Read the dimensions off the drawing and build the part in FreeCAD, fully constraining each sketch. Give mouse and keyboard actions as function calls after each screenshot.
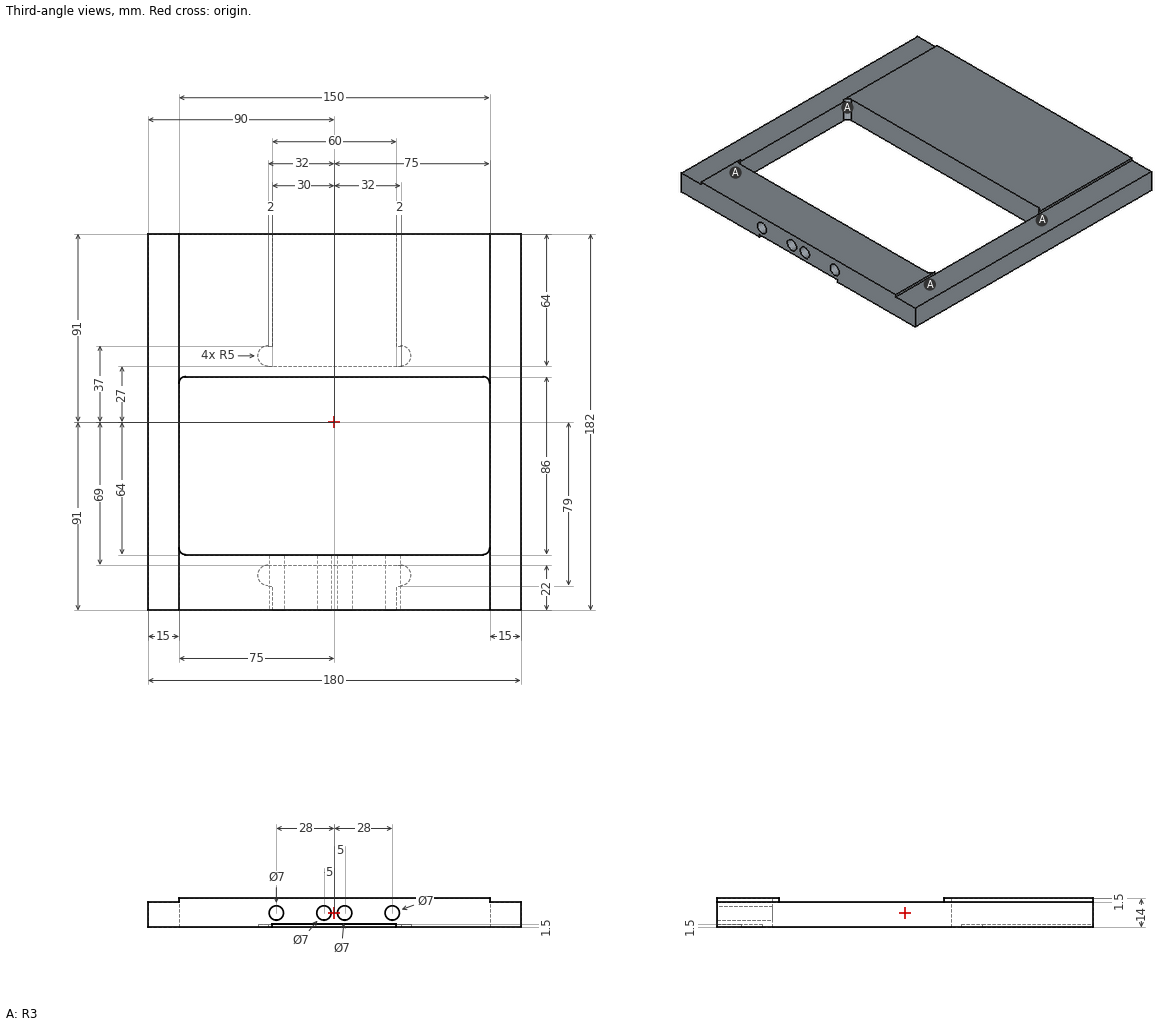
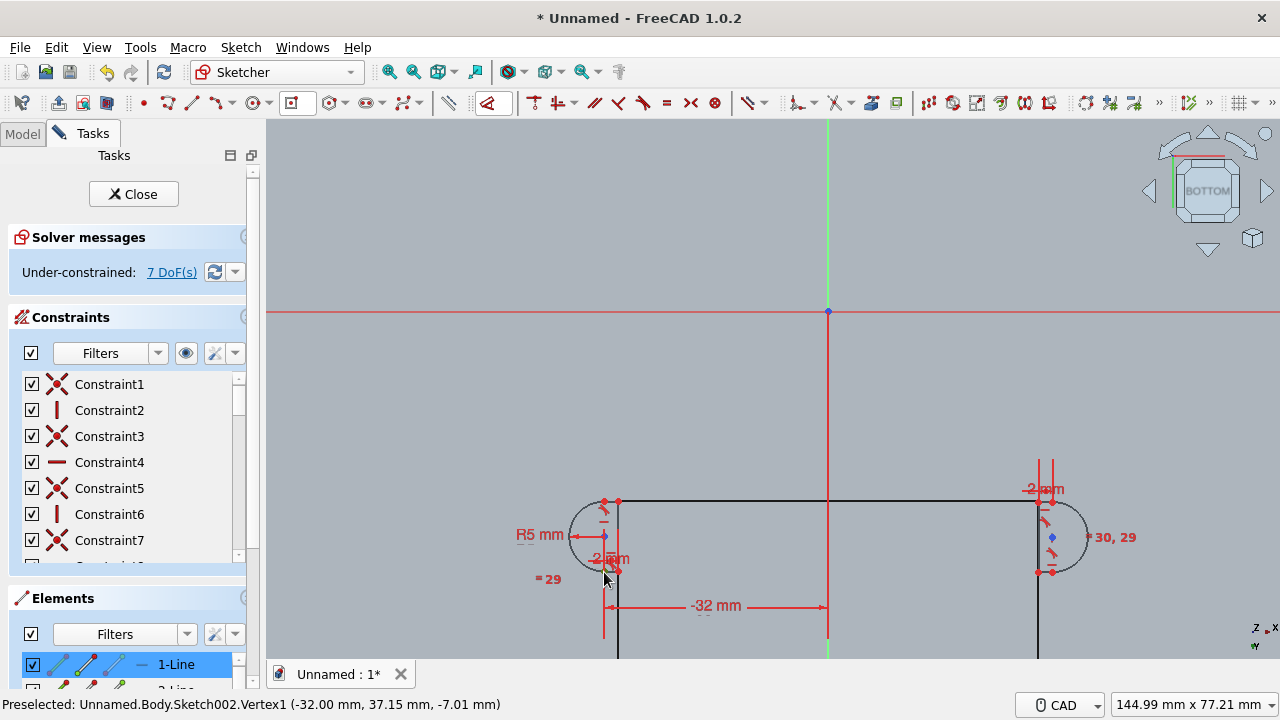
key(i)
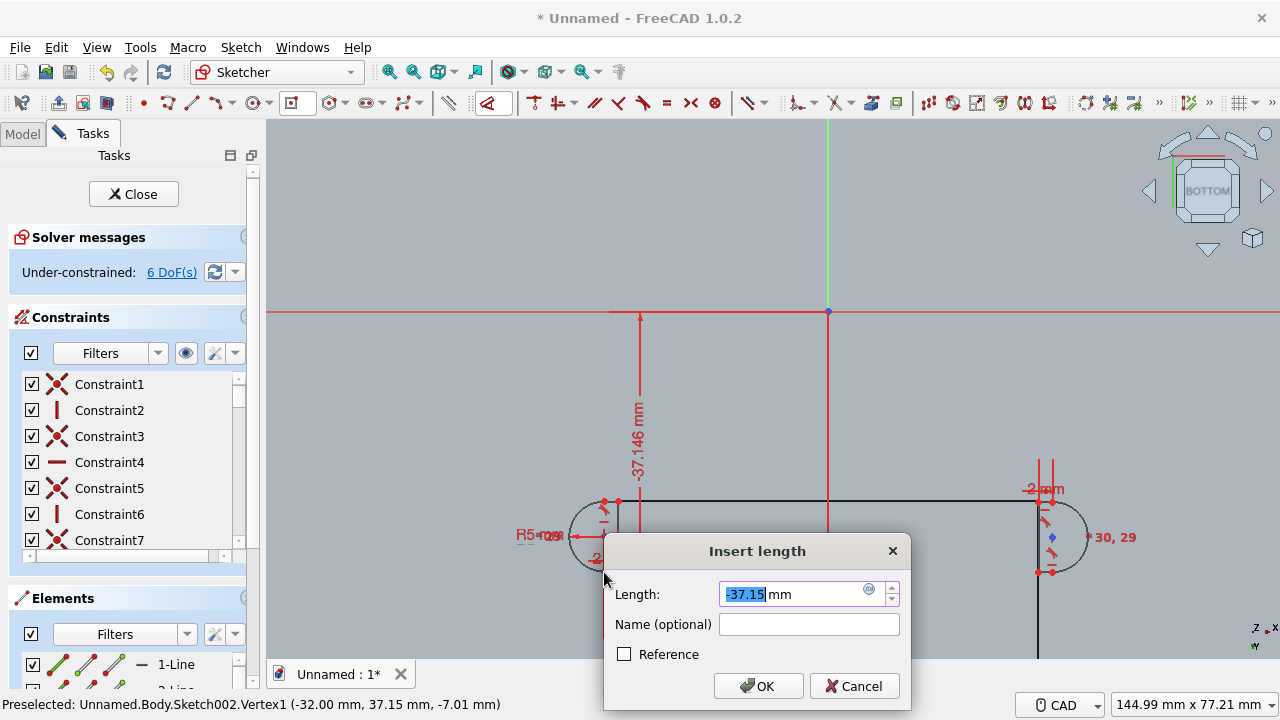
text(-37)
key(Return)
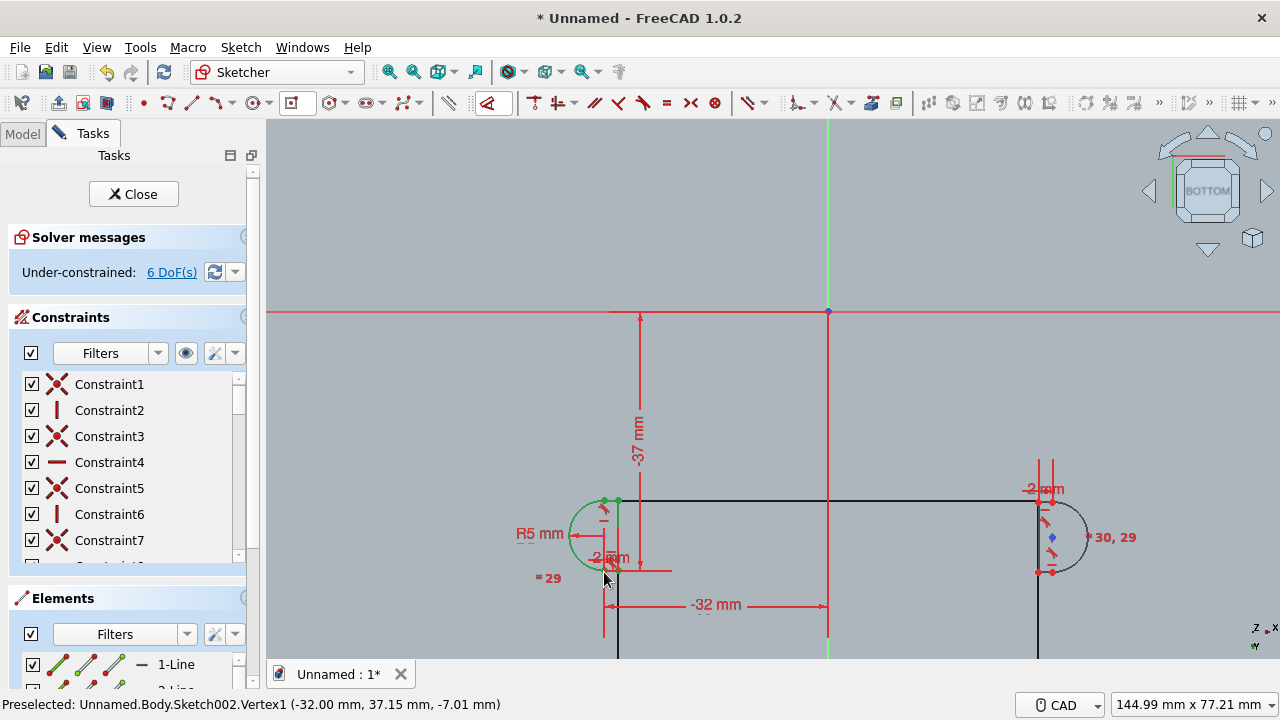
click(1053, 502)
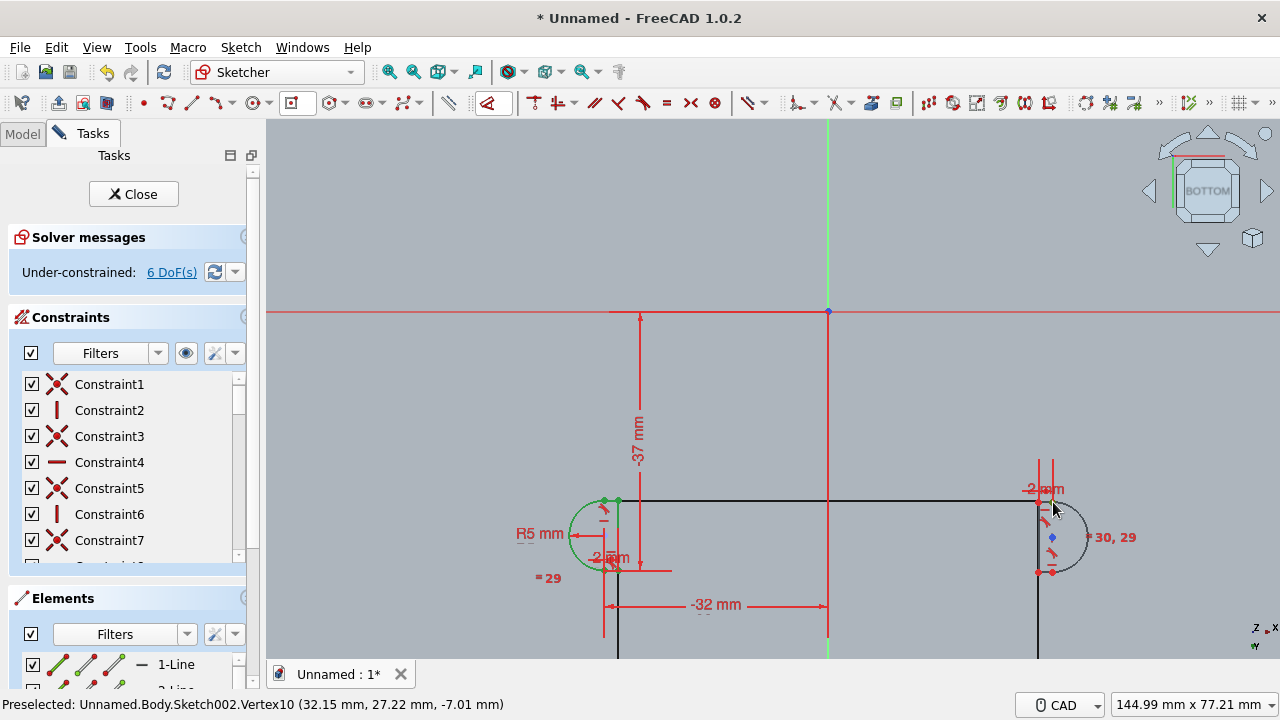
key(l)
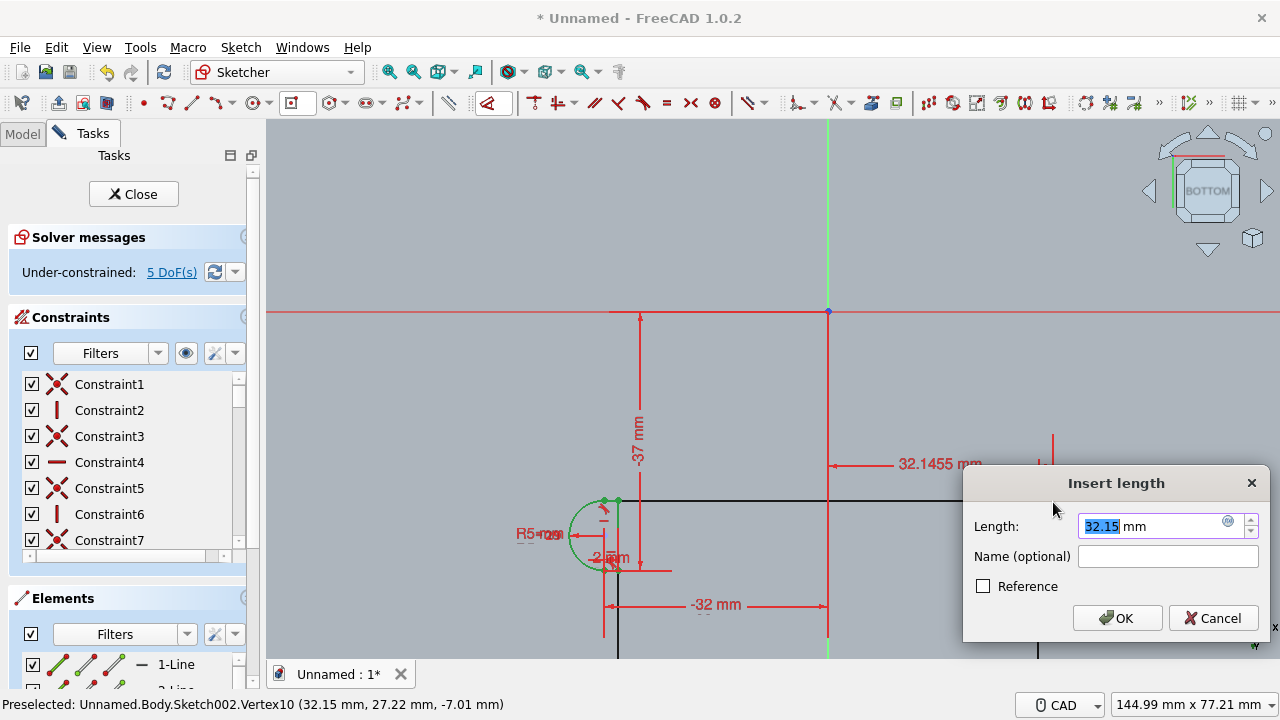
text(32)
key(Return)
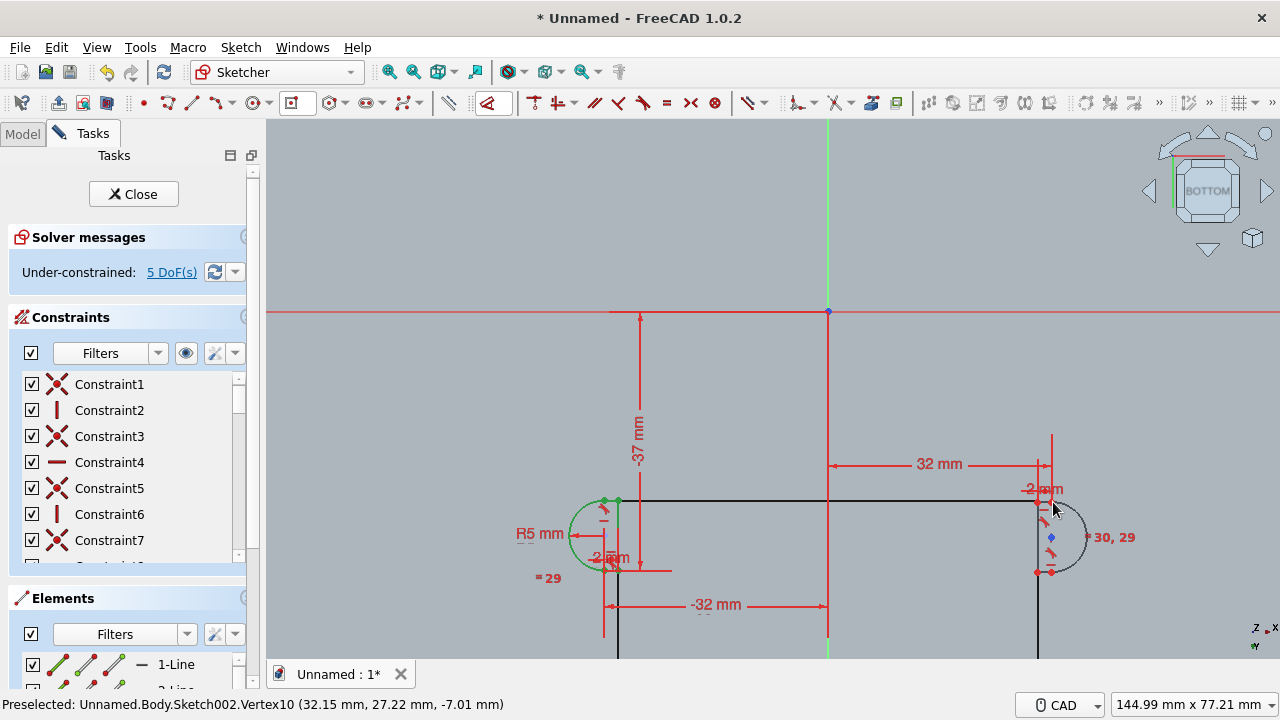
click(1052, 502)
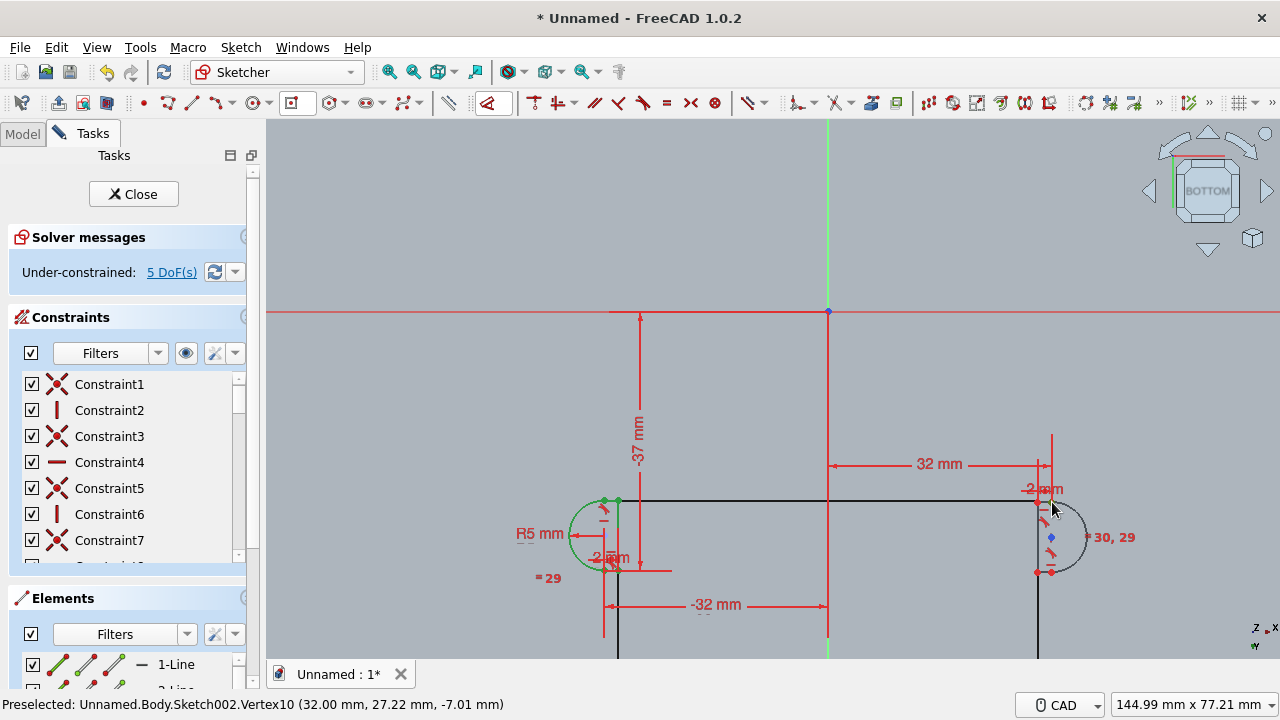
click(506, 104)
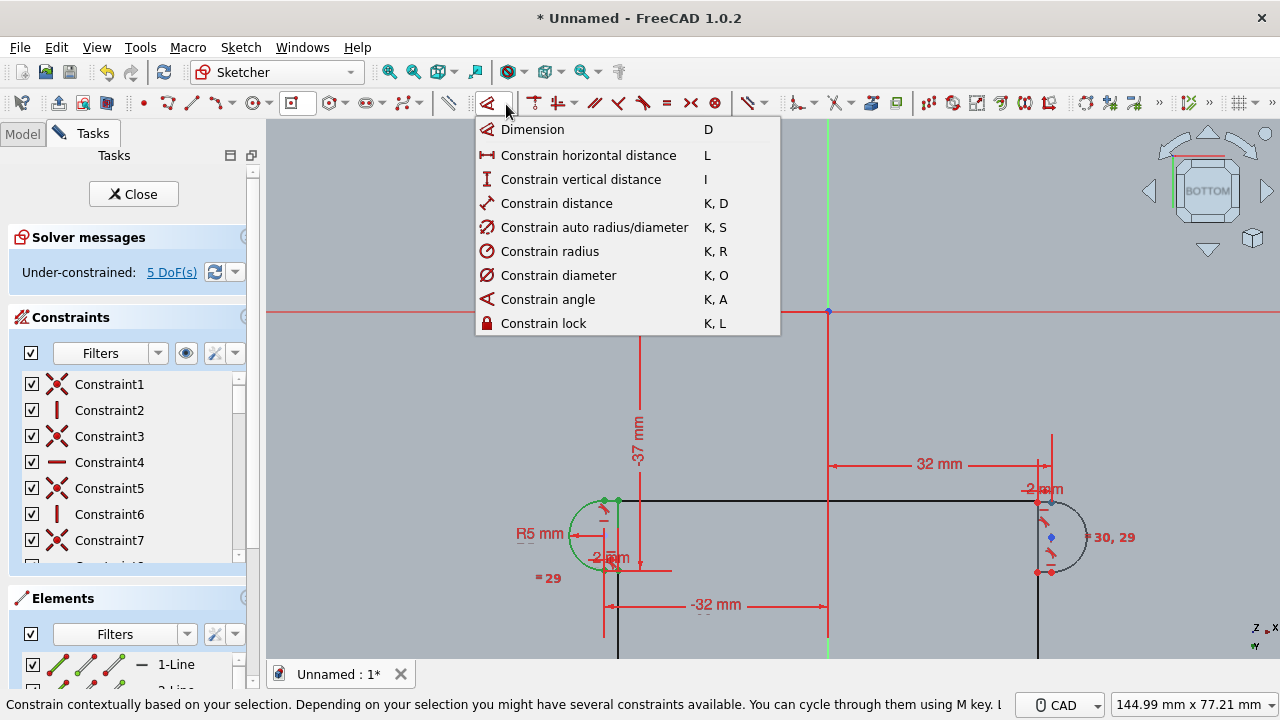
click(628, 179)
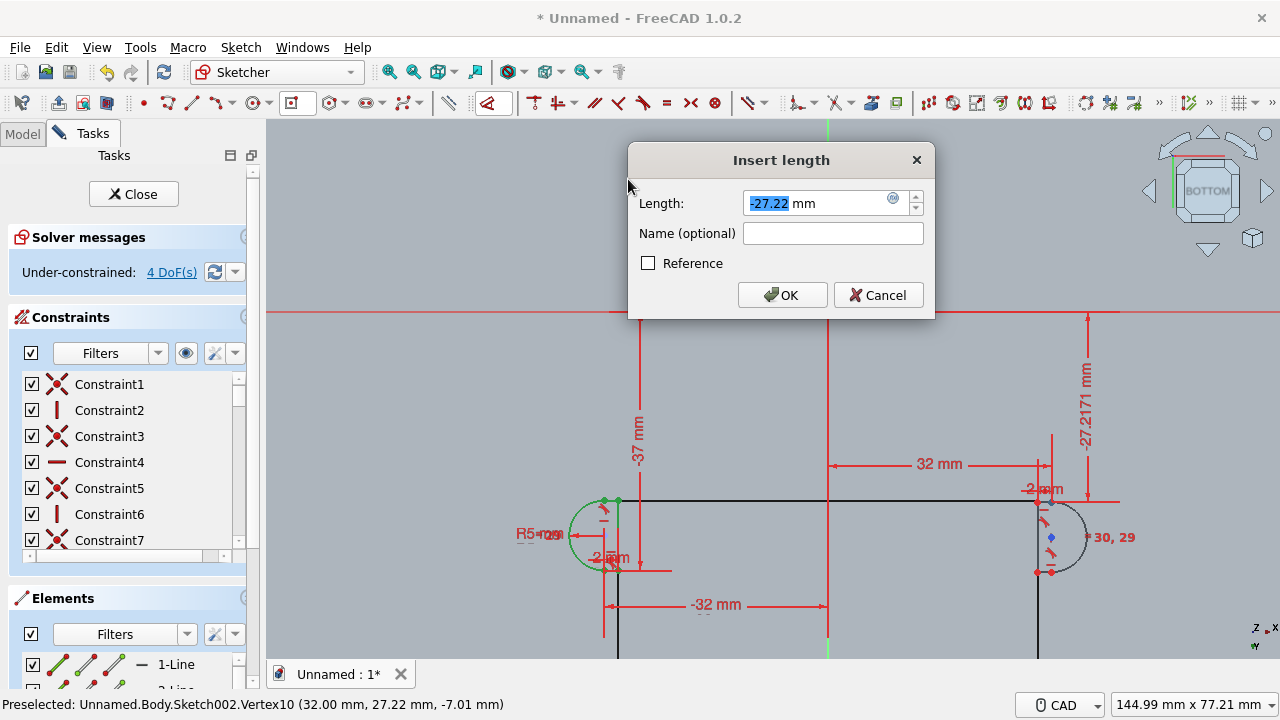
text(-27)
key(Return)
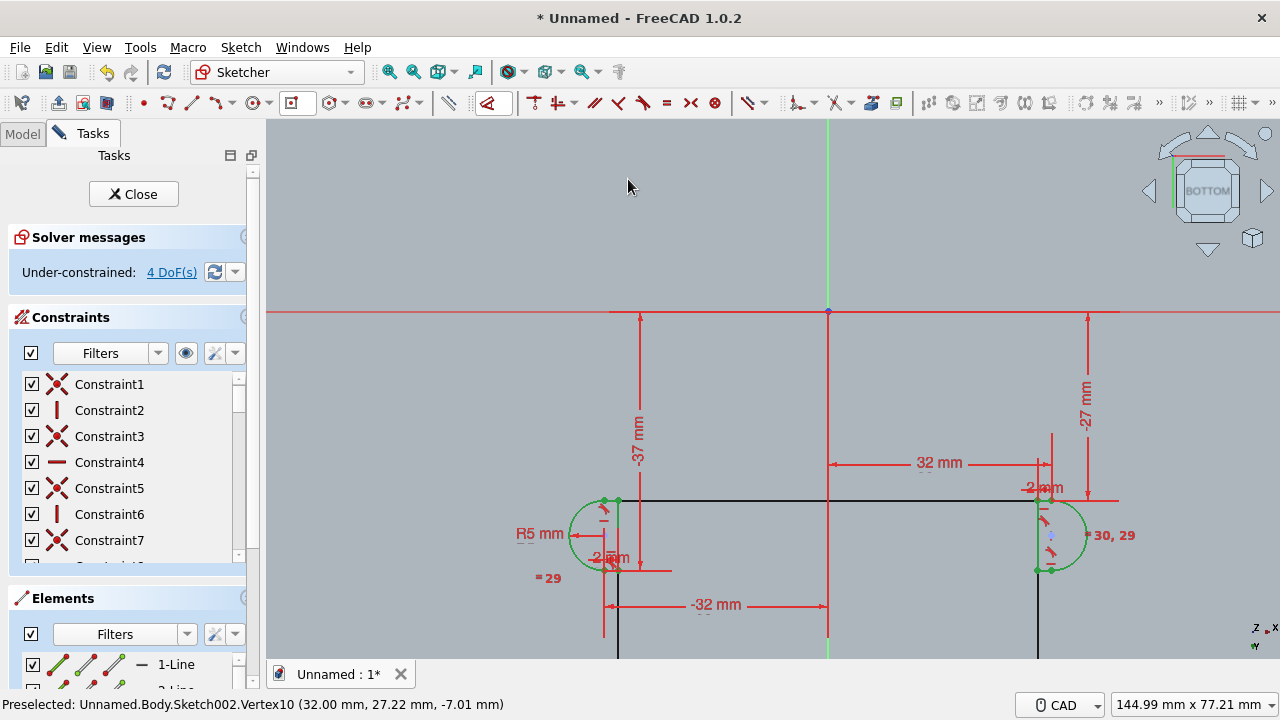
scroll(604, 572, down, 4)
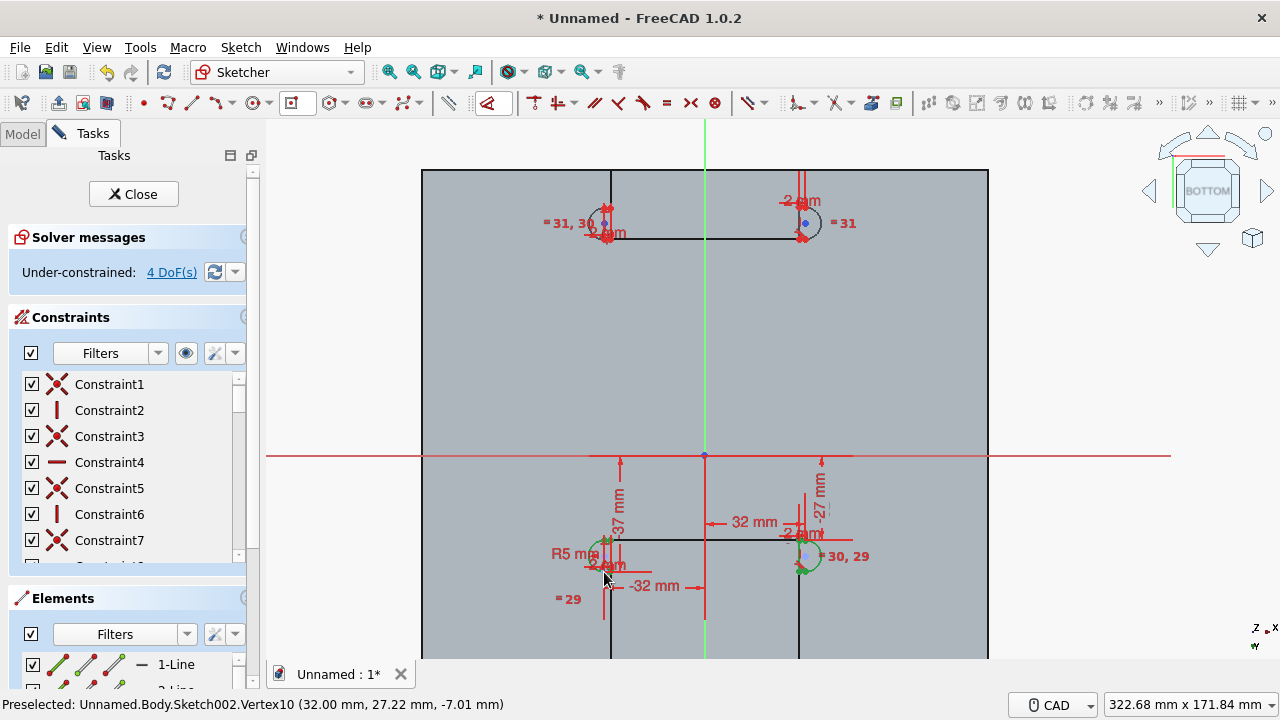
scroll(604, 240, up, 4)